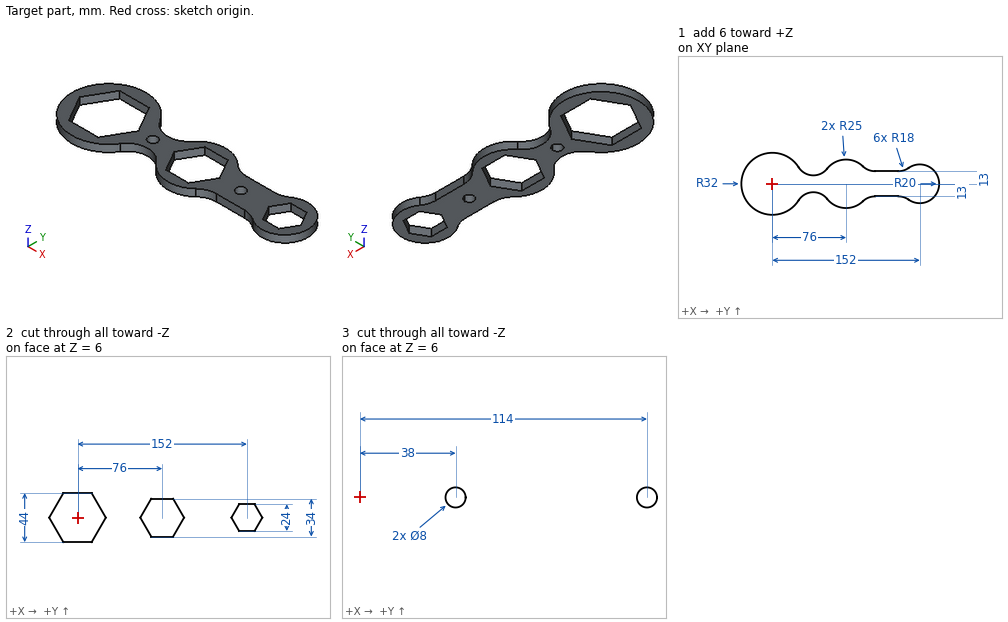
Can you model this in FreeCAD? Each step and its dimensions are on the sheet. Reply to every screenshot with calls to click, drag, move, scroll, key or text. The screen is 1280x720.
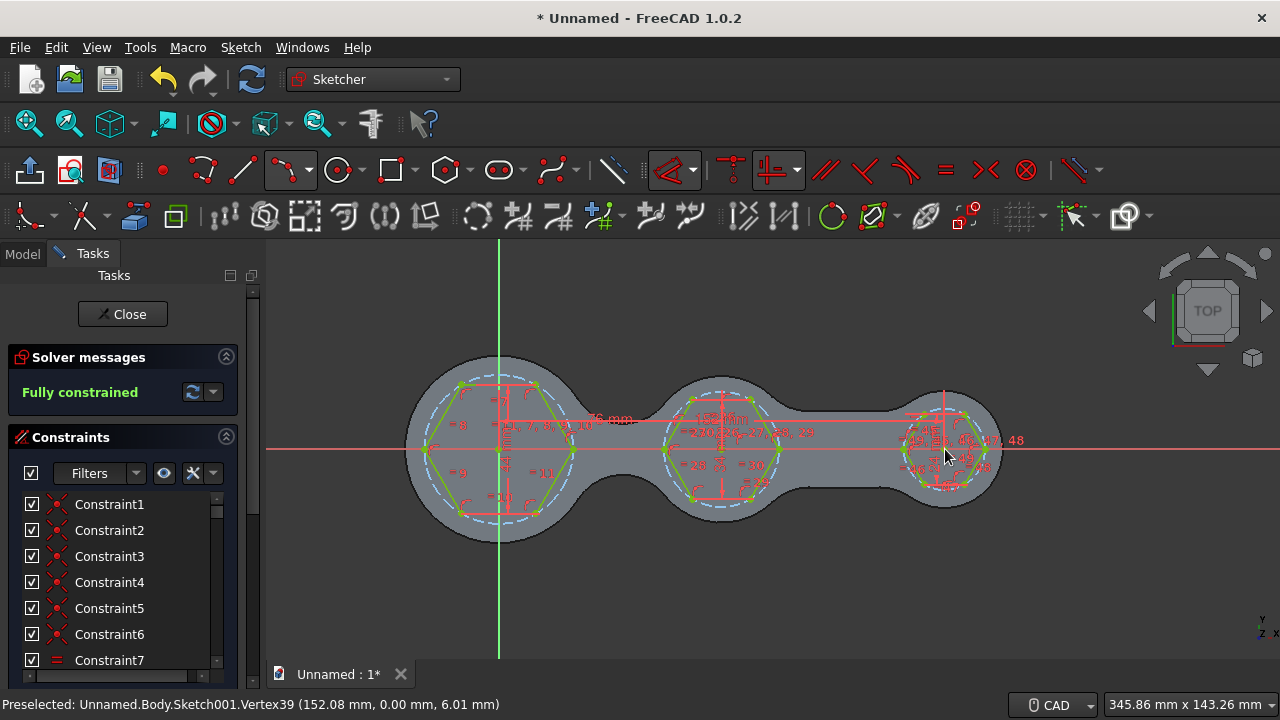
click(123, 314)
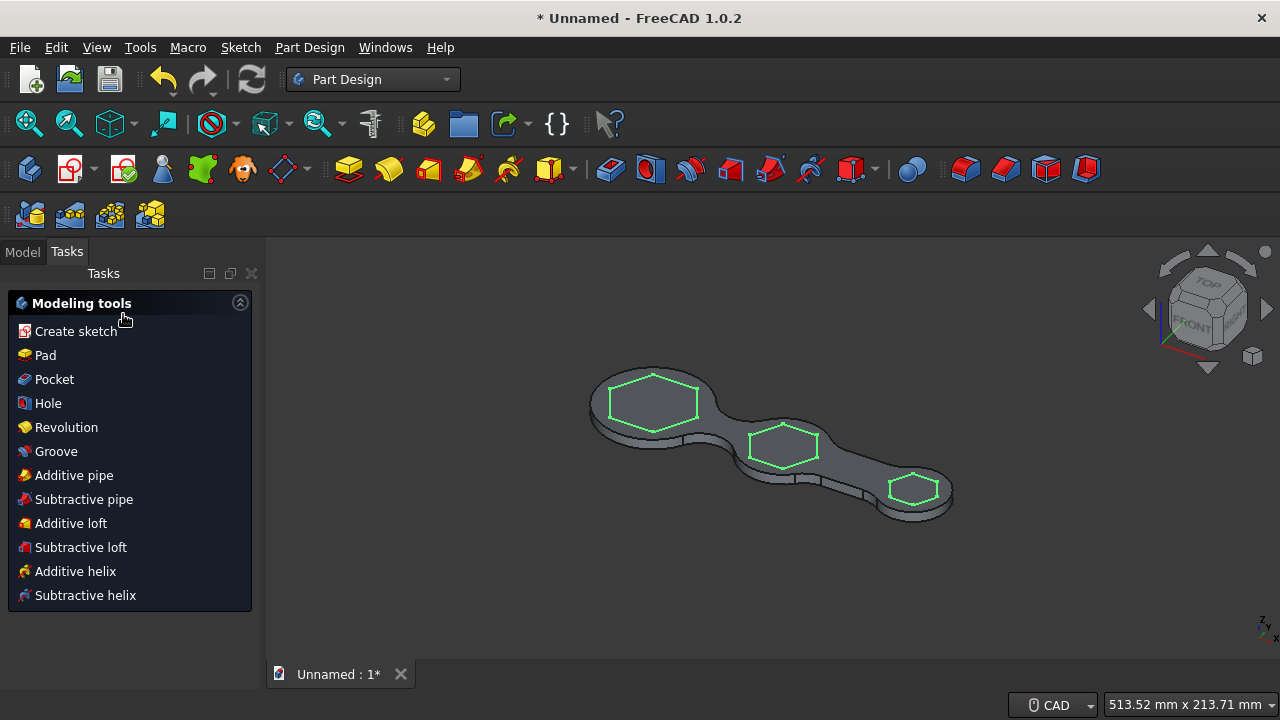
click(612, 170)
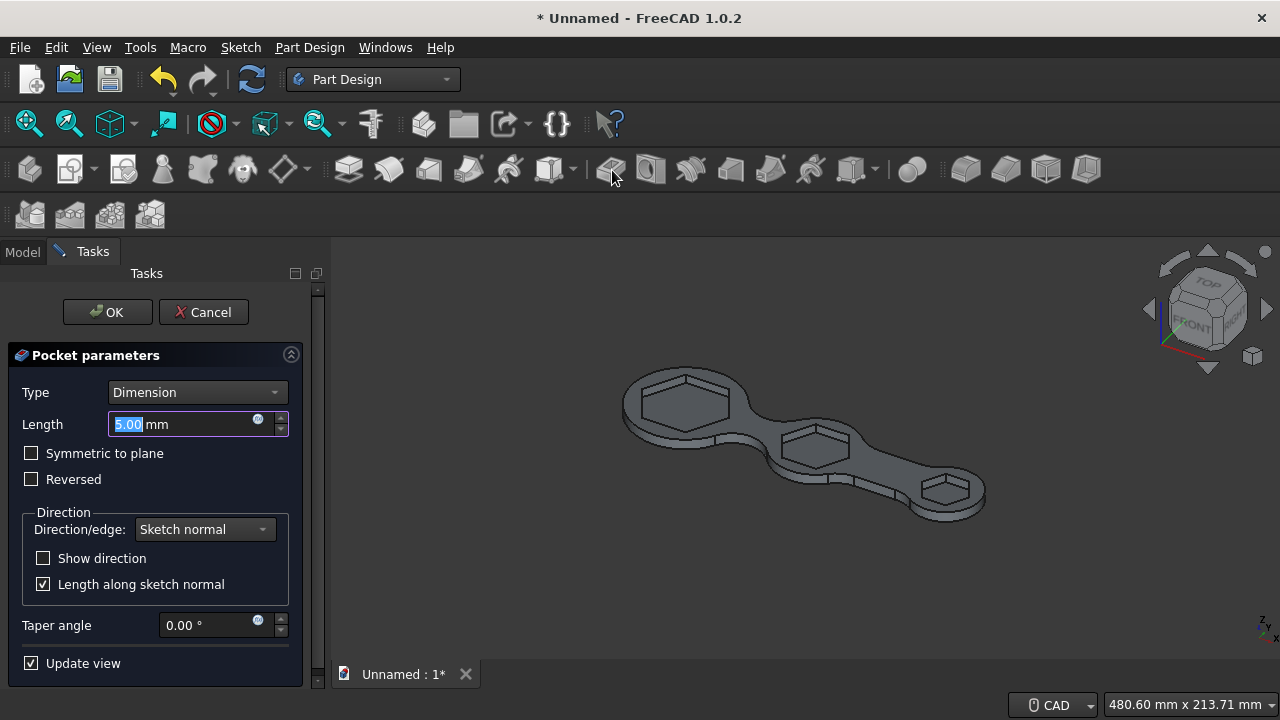
click(198, 392)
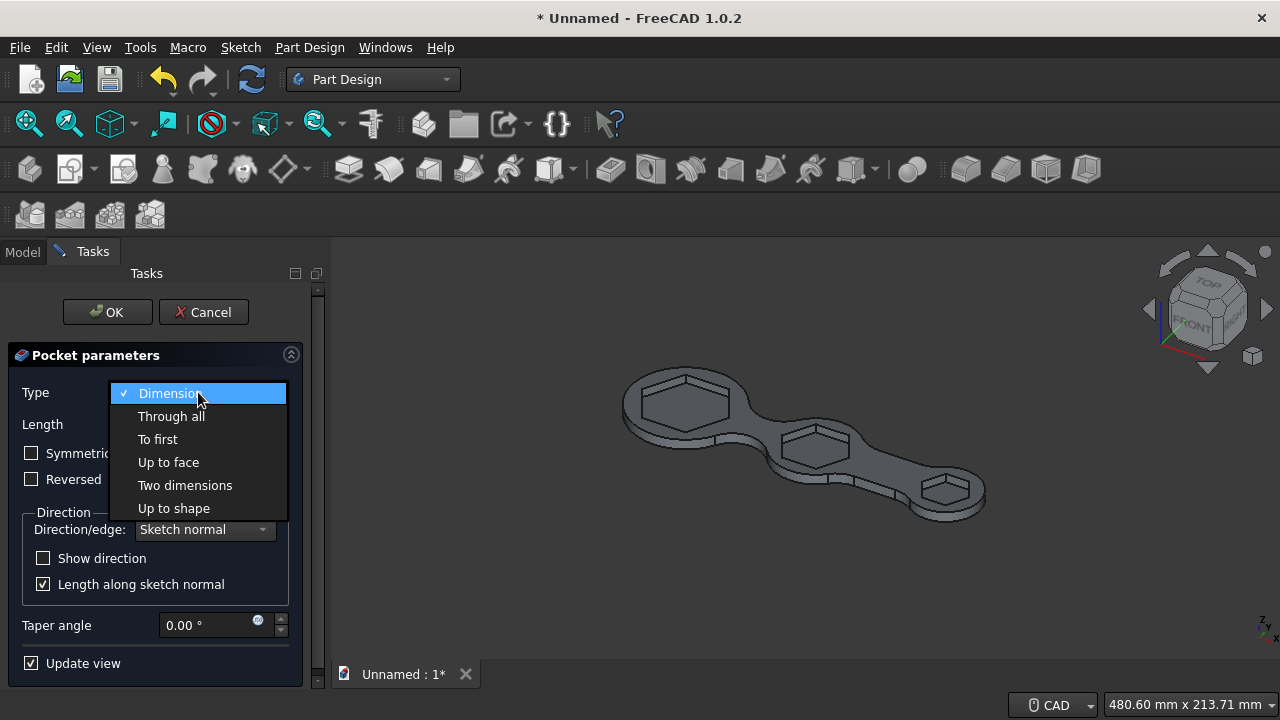
click(198, 416)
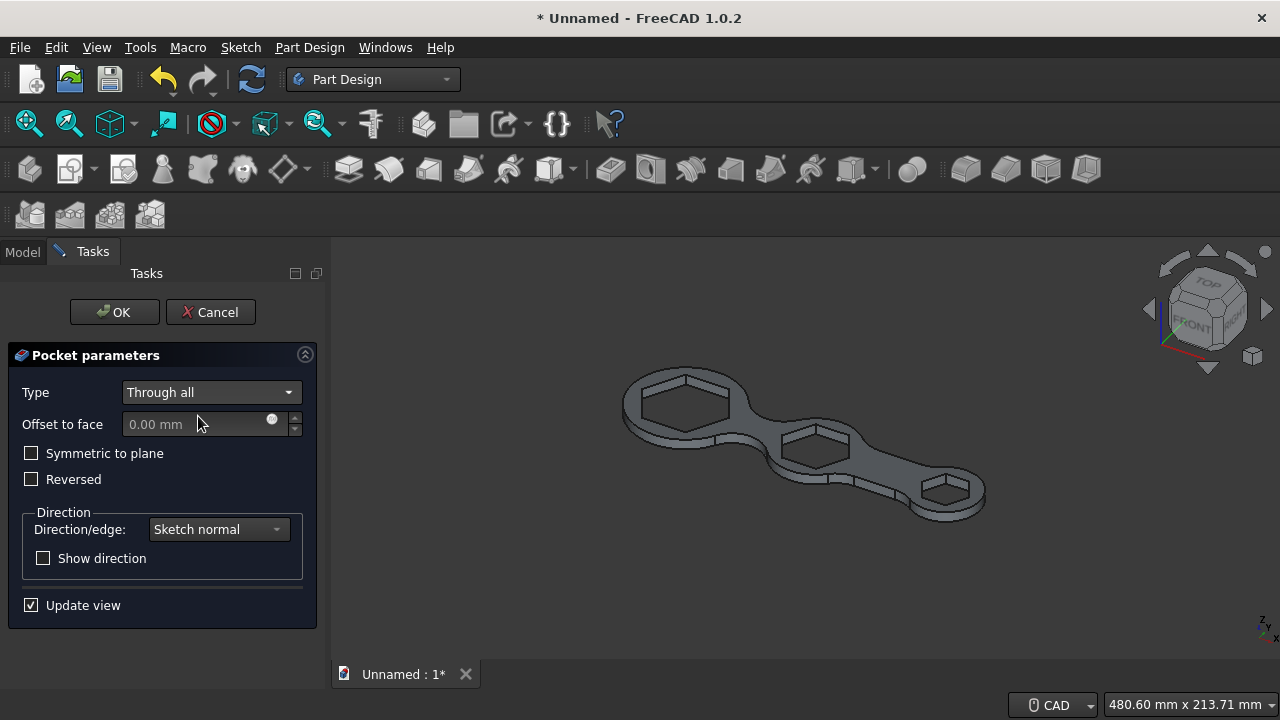
click(115, 312)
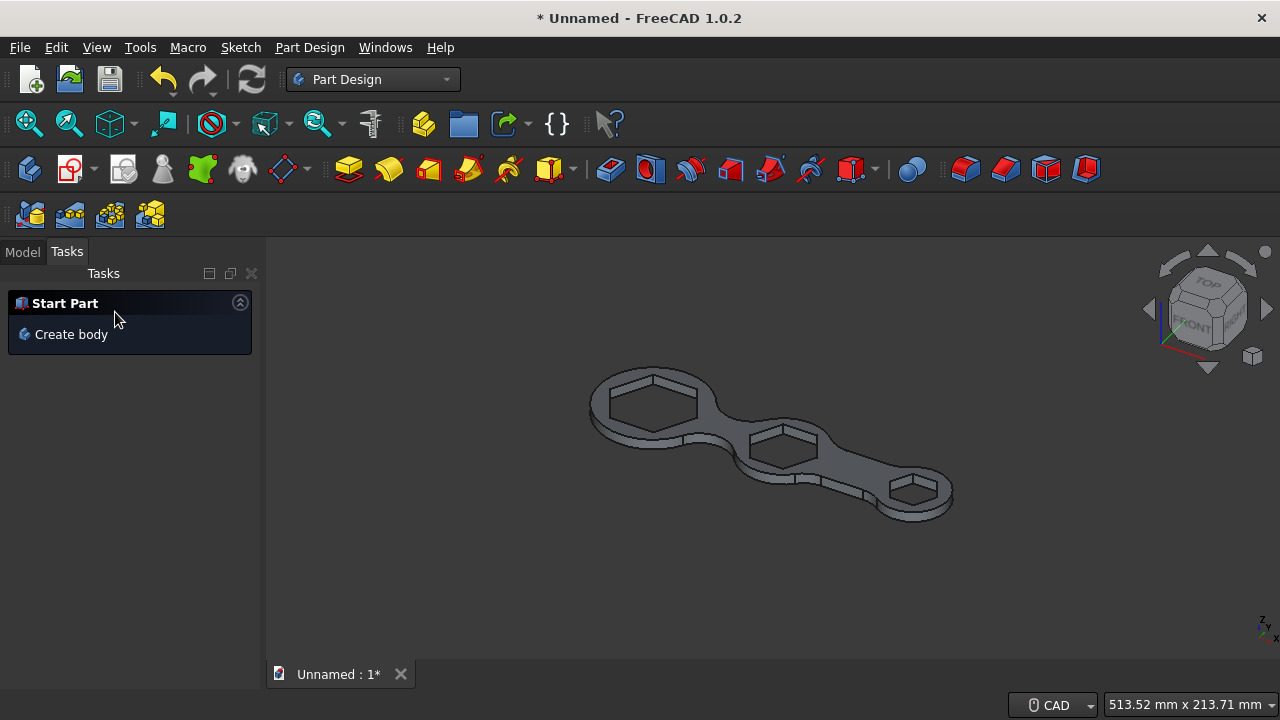
click(30, 124)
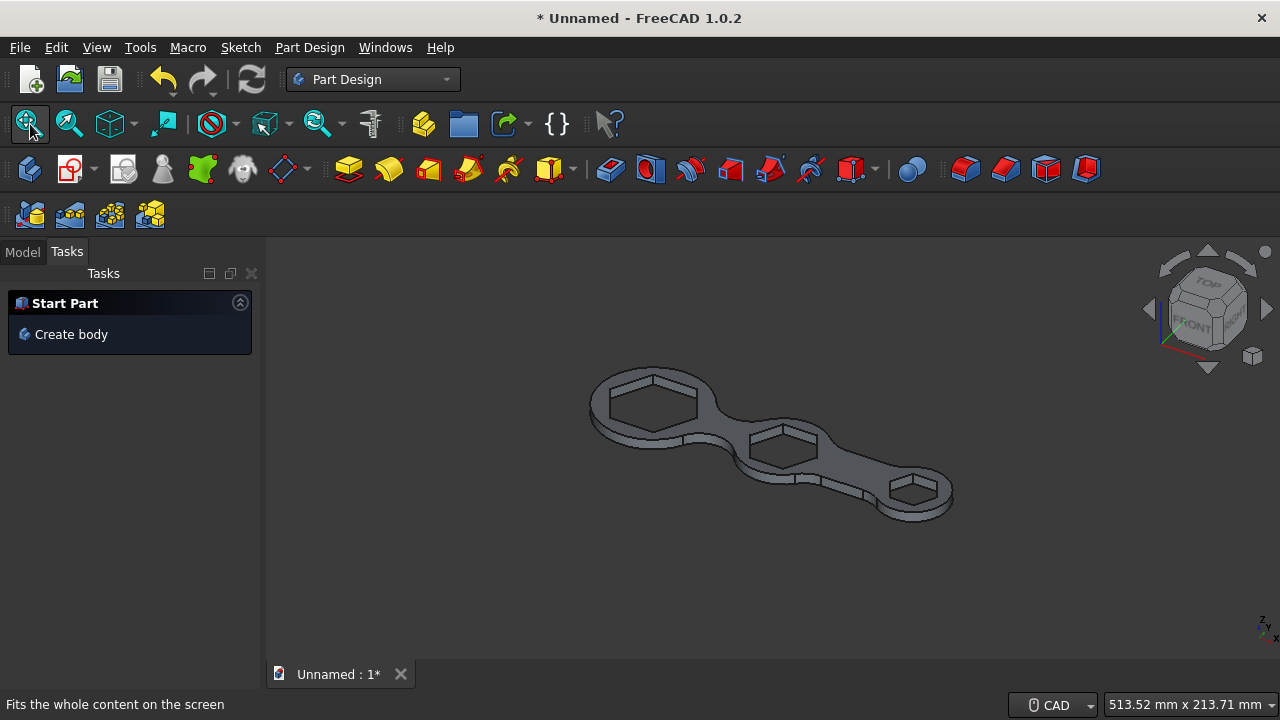
click(873, 475)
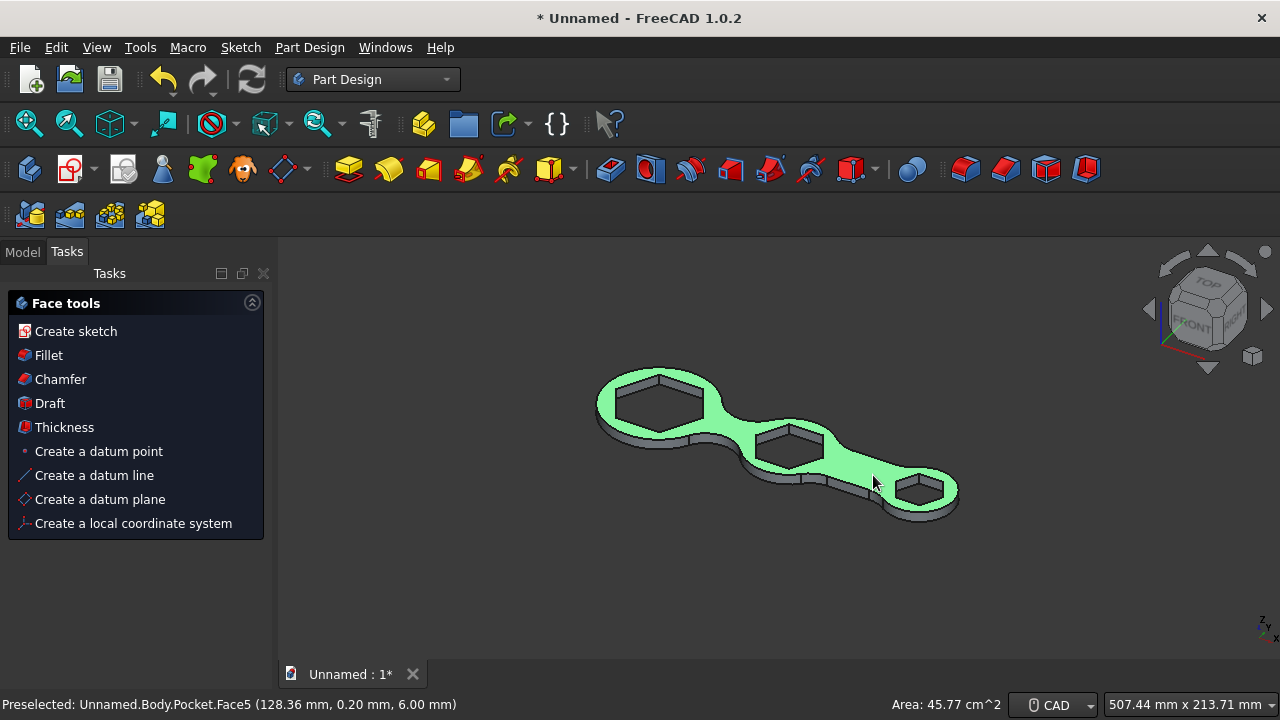
click(70, 170)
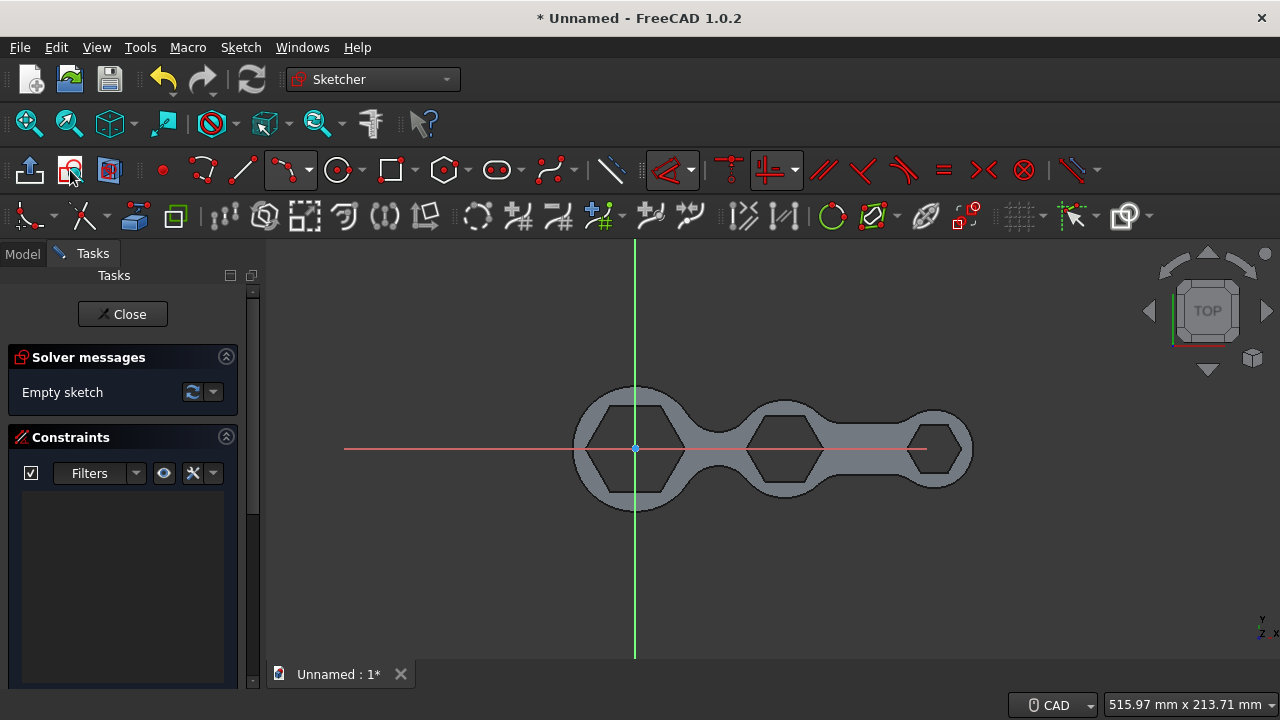
scroll(779, 449, up, 5)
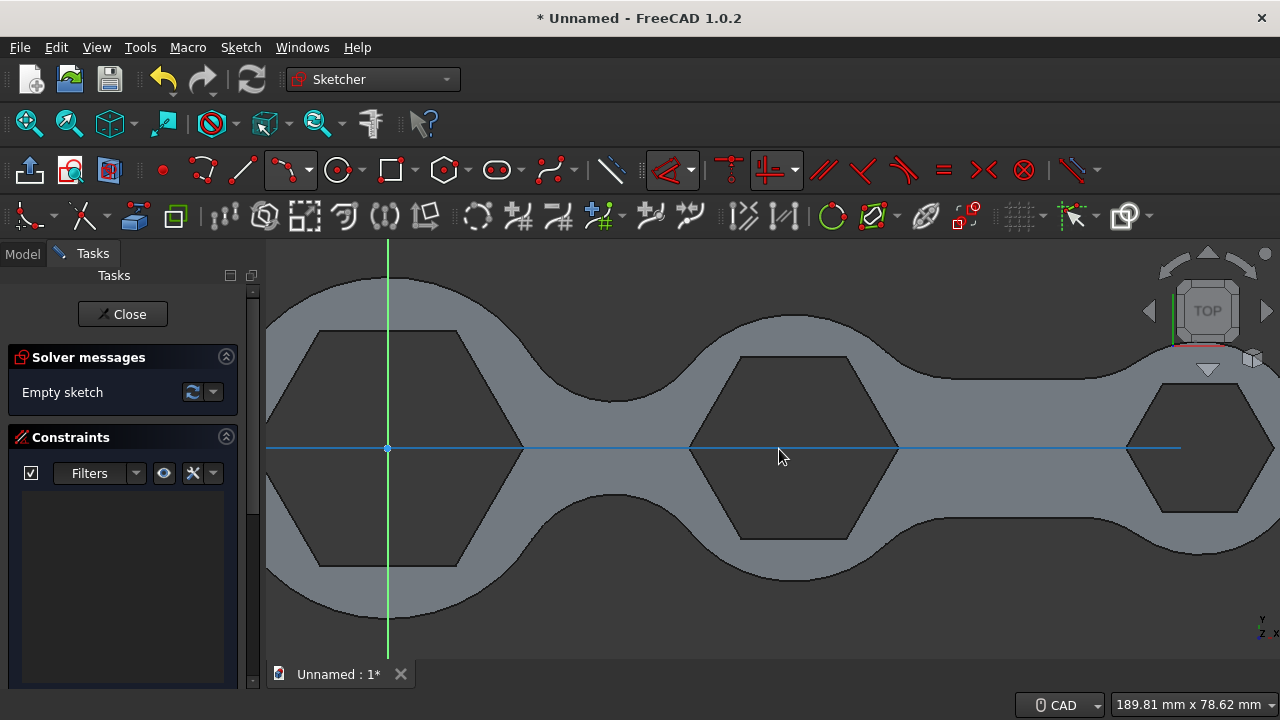
click(338, 170)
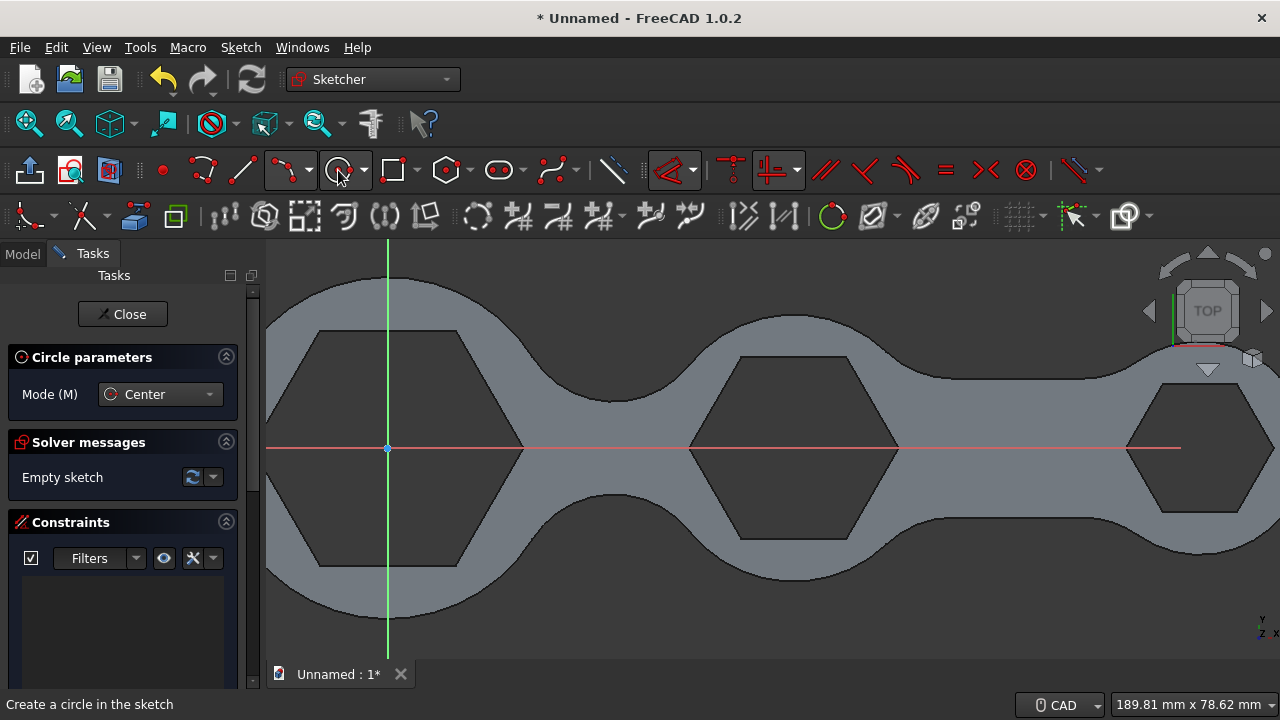
click(591, 448)
move(606, 433)